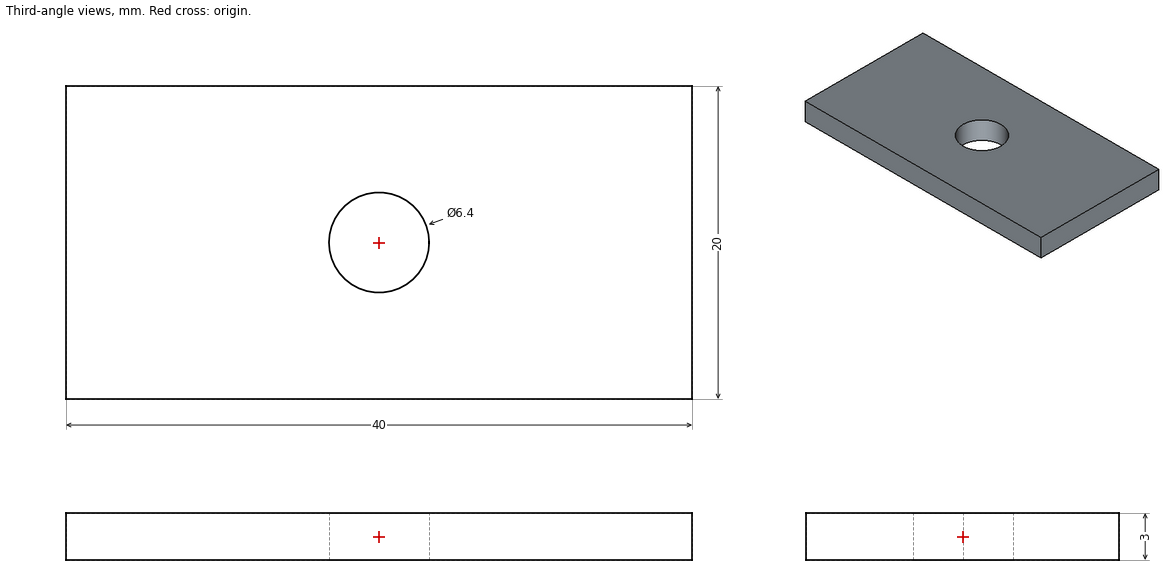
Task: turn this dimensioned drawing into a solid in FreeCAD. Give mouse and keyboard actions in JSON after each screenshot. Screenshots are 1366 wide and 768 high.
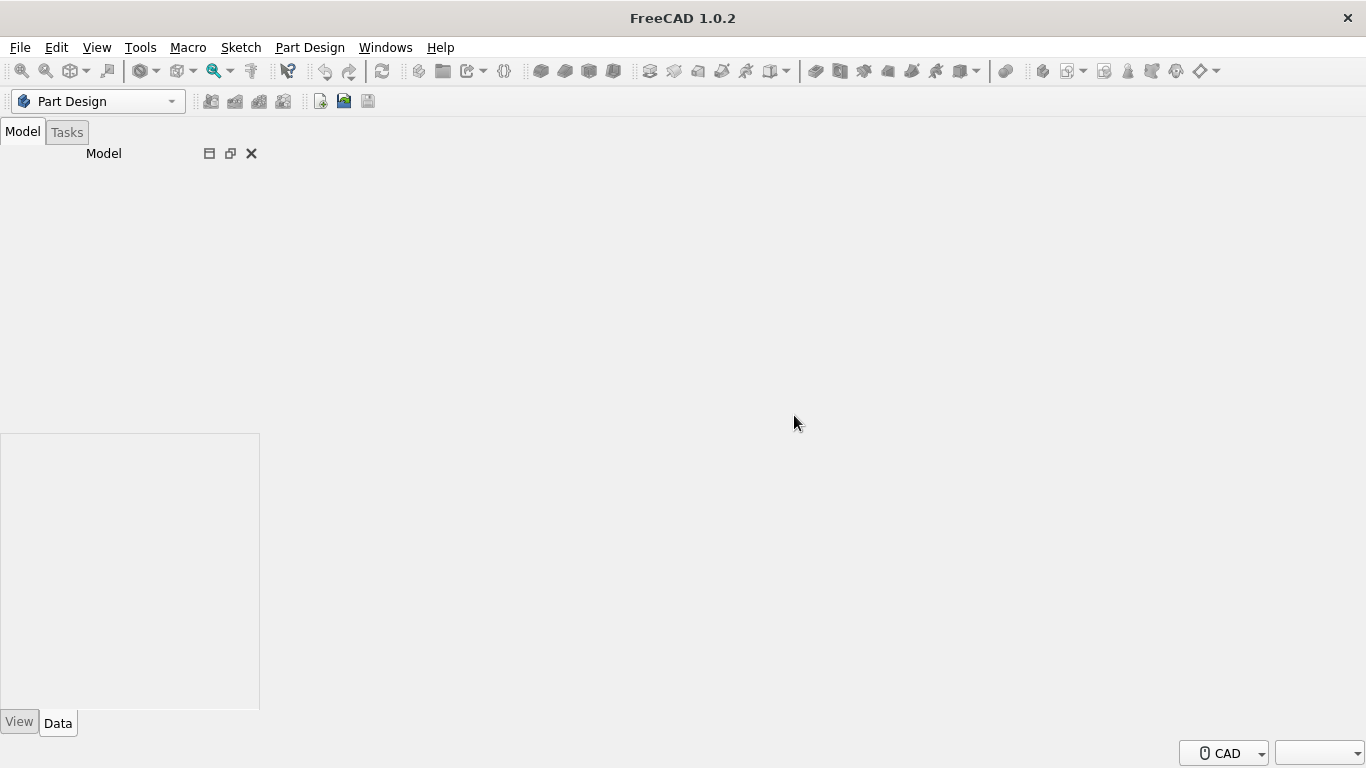
{"action": "left_click", "coordinate": [320, 102]}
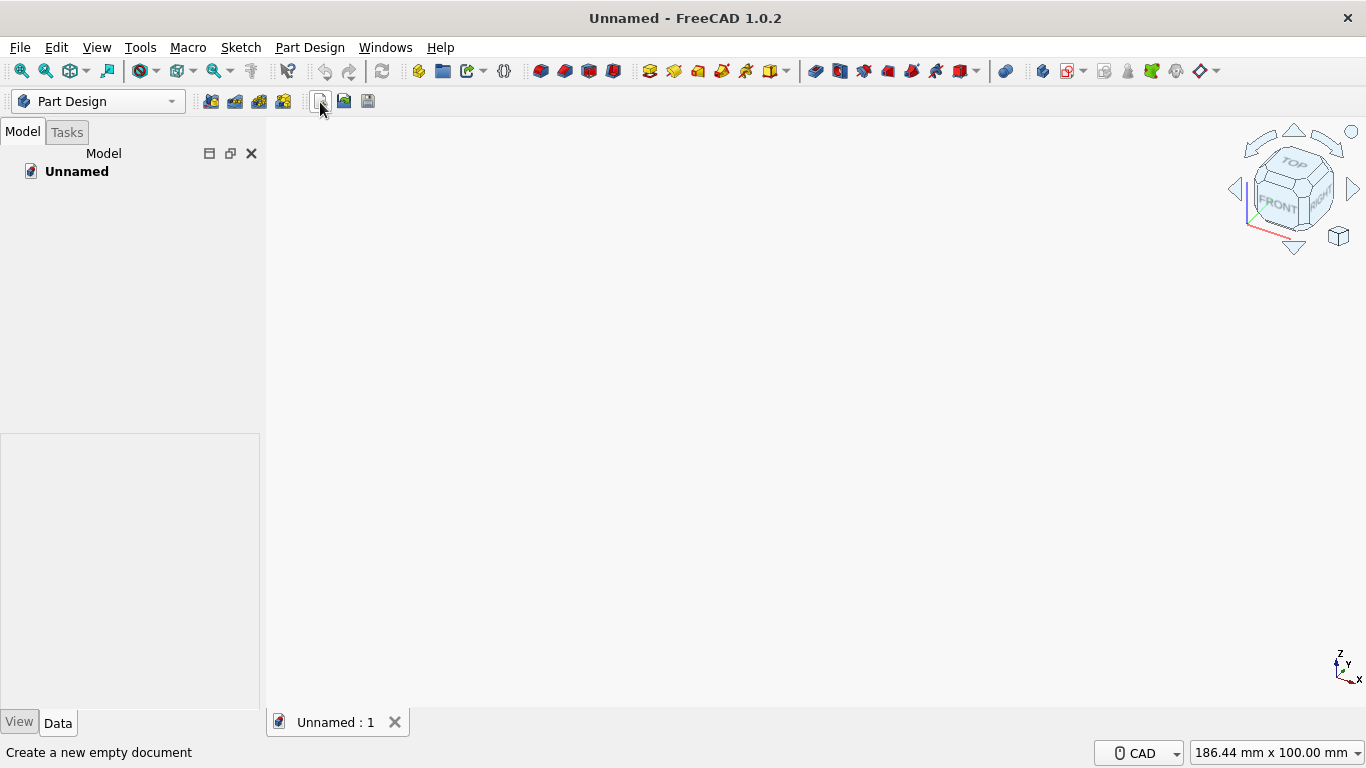
{"action": "left_click", "coordinate": [1068, 72]}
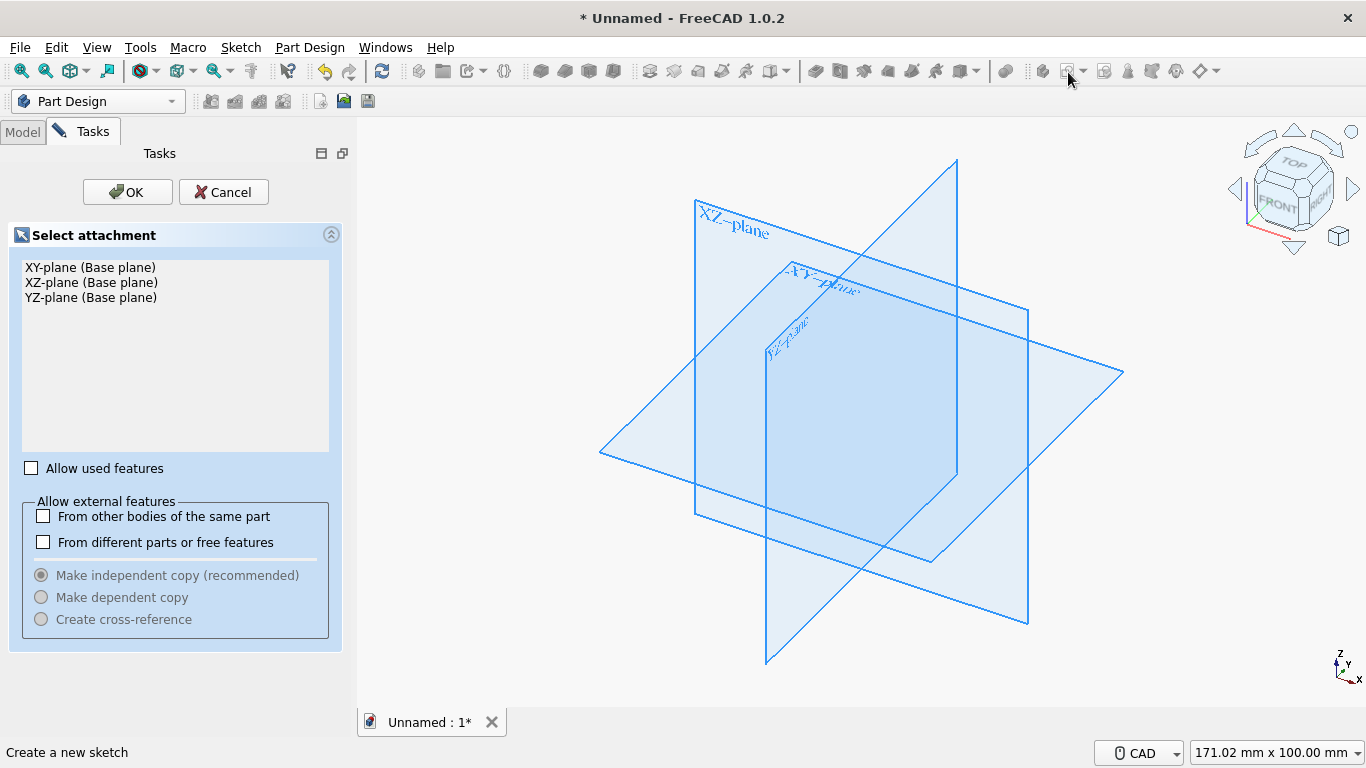
{"action": "left_click", "coordinate": [82, 268]}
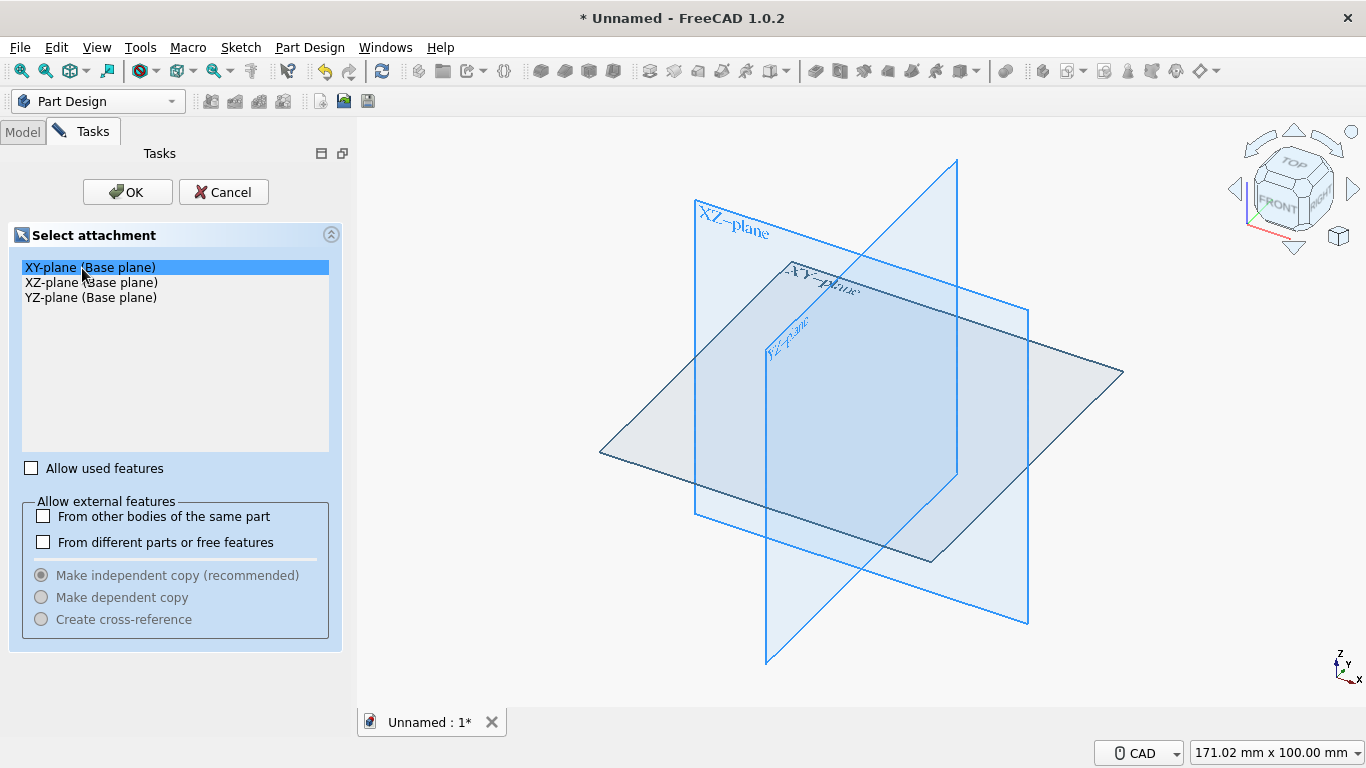
{"action": "left_click", "coordinate": [128, 192]}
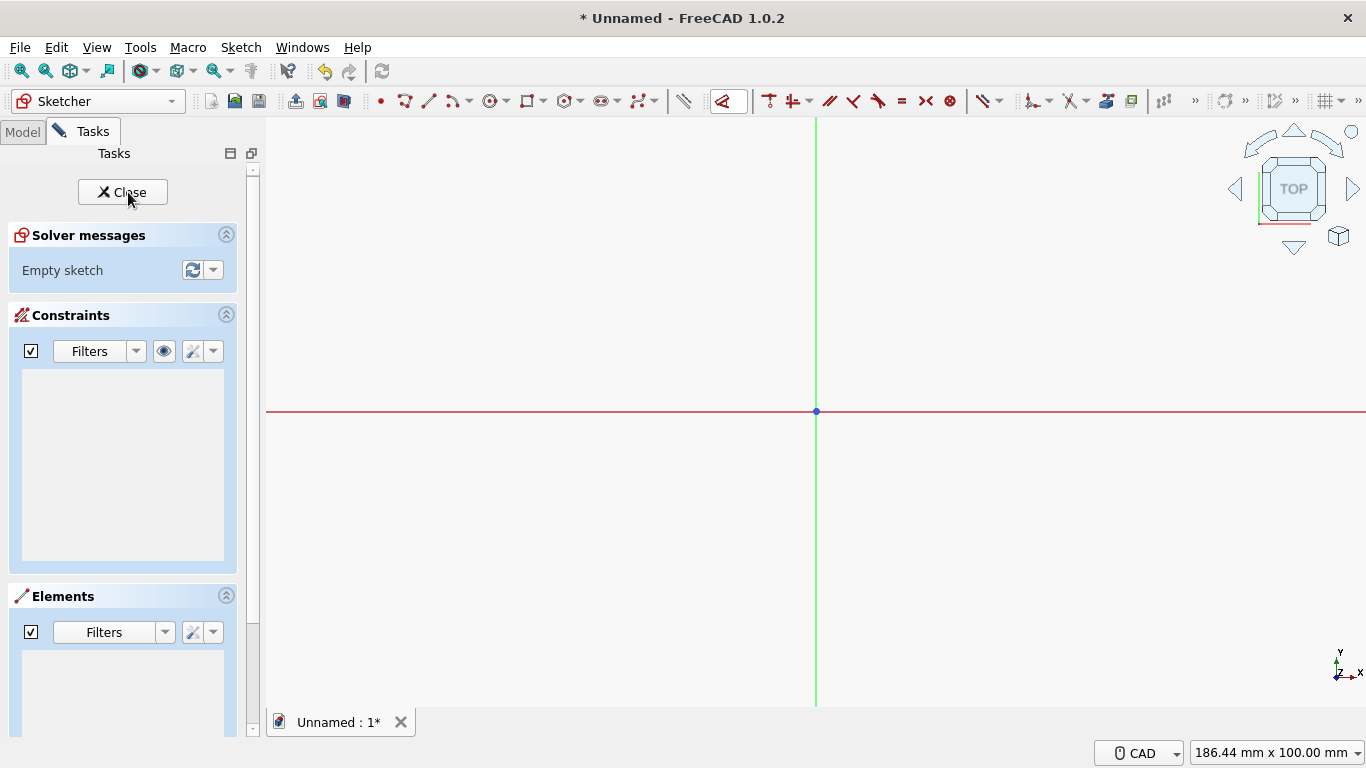
{"action": "scroll", "coordinate": [856, 412], "scroll_direction": "up", "scroll_amount": 5}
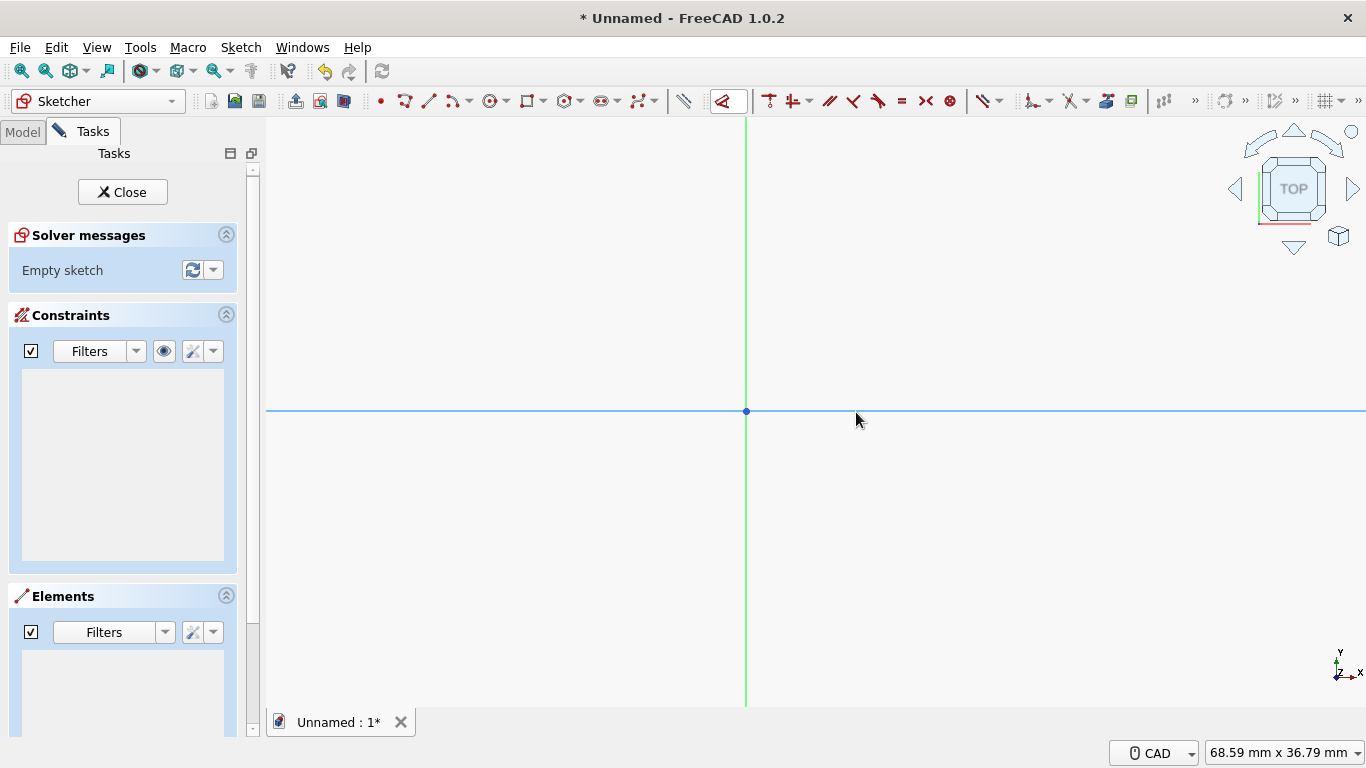
{"action": "key", "text": "g v"}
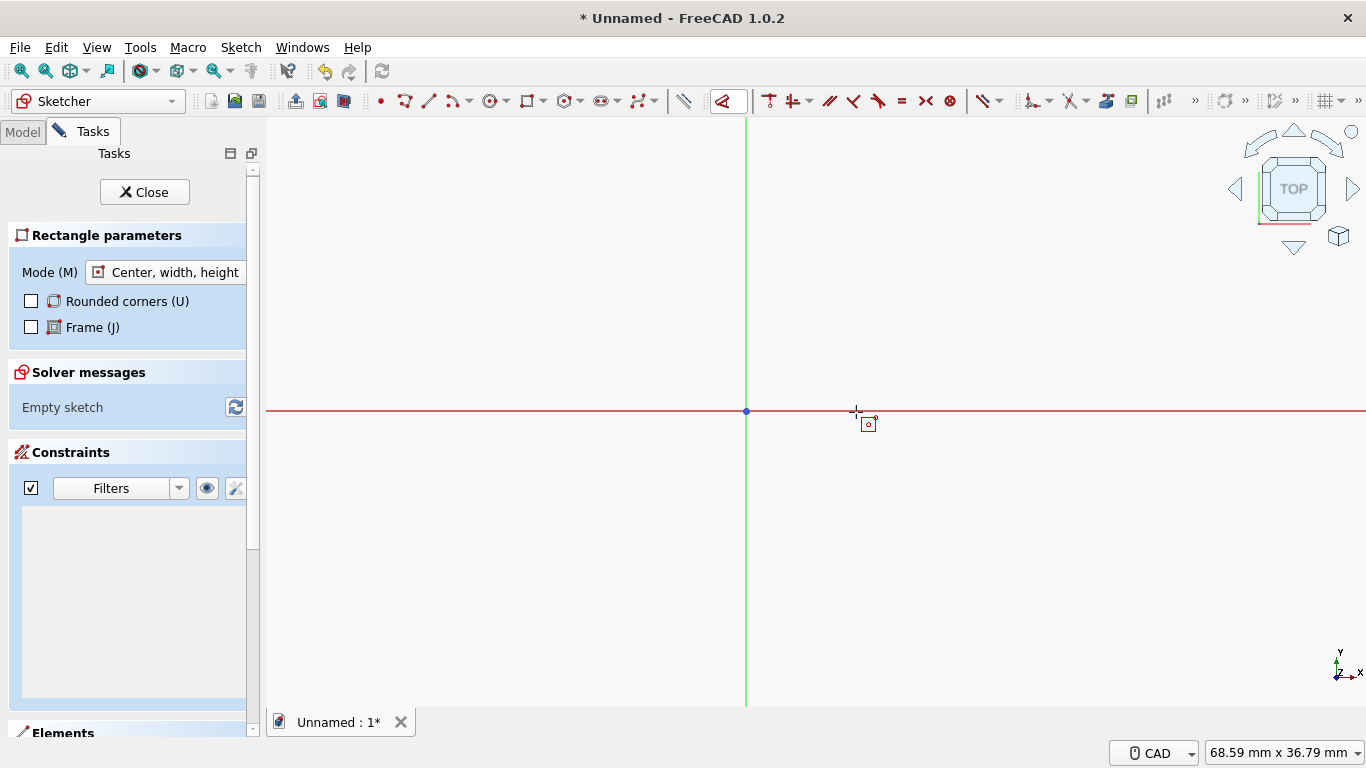
{"action": "left_click", "coordinate": [746, 411]}
{"action": "left_click", "coordinate": [1067, 251]}
{"action": "key", "text": "Escape"}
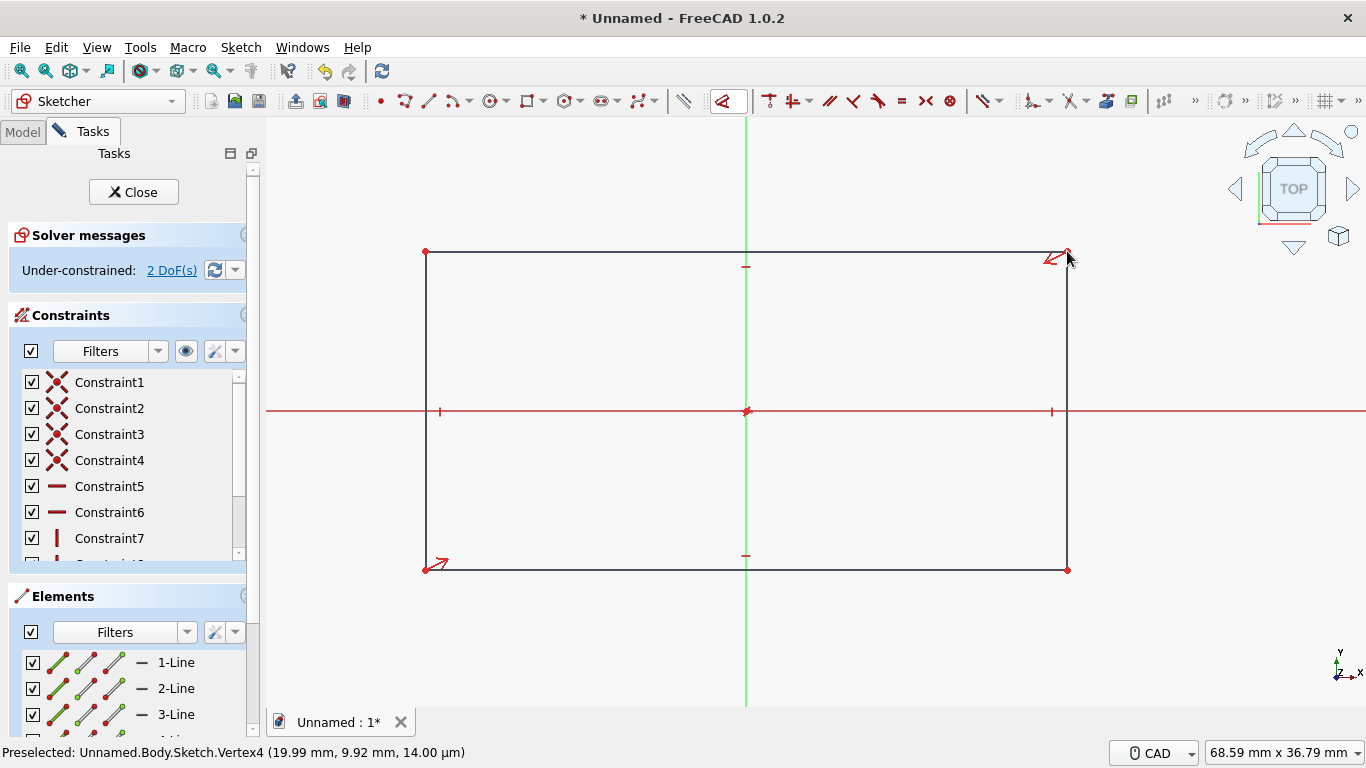
{"action": "left_click", "coordinate": [722, 102]}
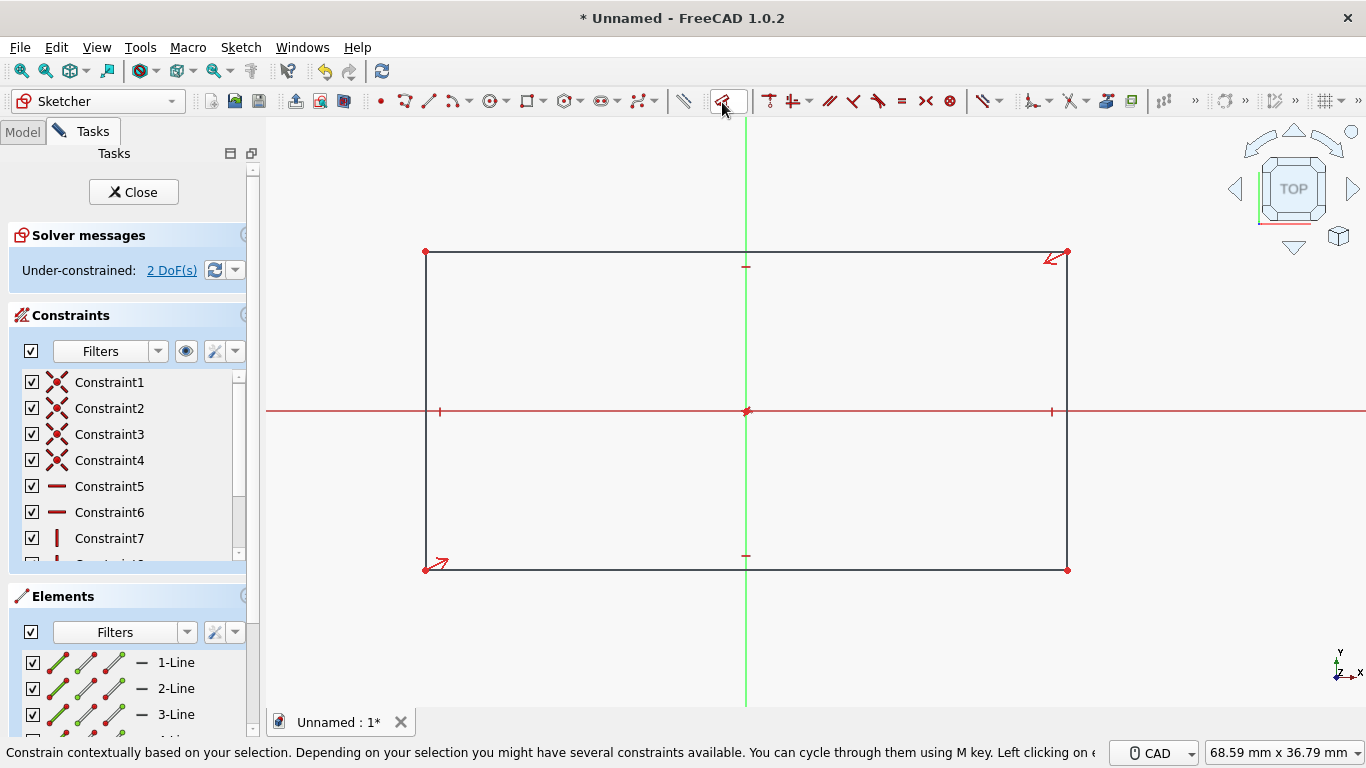
{"action": "left_click", "coordinate": [618, 570]}
{"action": "left_click", "coordinate": [599, 604]}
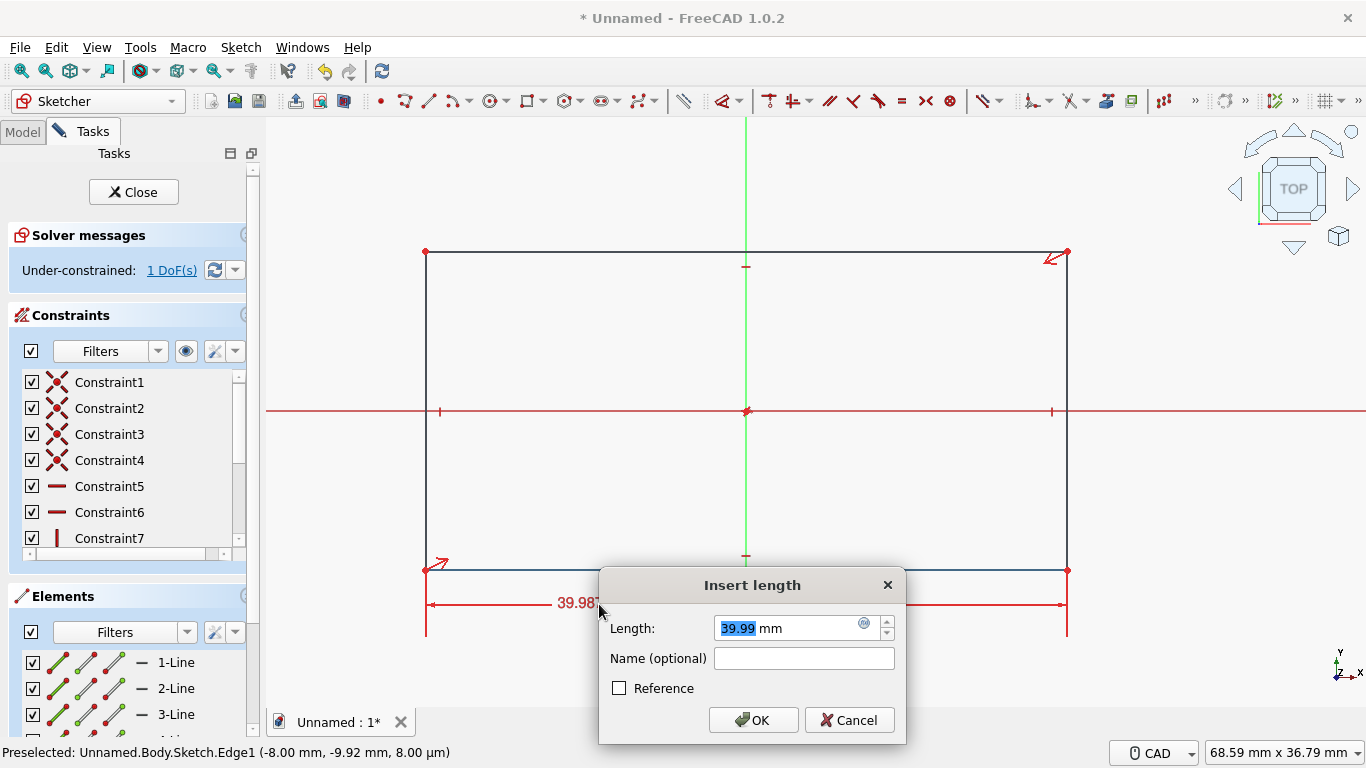
{"action": "type", "text": "40"}
{"action": "key", "text": "Return"}